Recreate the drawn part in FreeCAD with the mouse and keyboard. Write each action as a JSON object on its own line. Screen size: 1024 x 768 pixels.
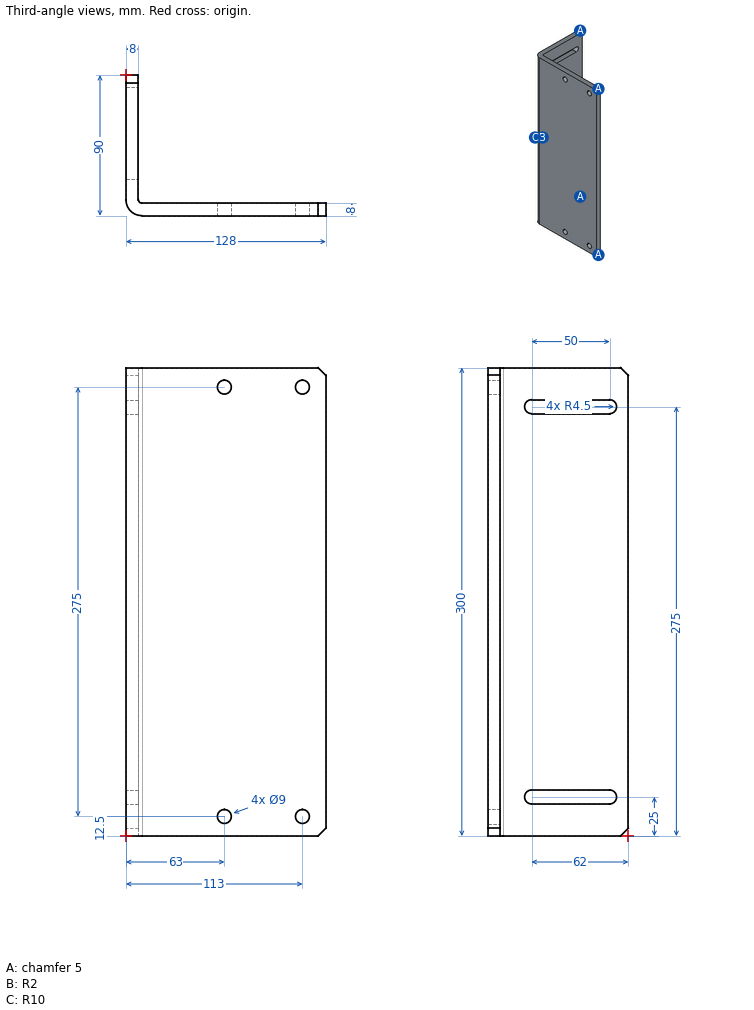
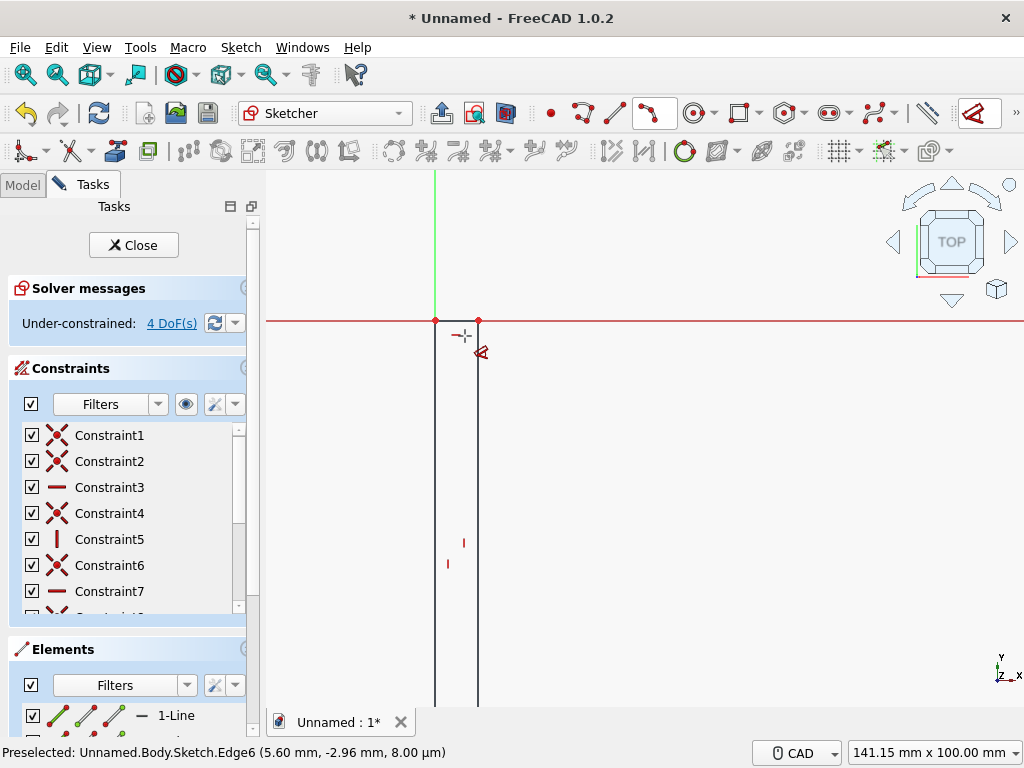
{"action": "scroll", "coordinate": [330, 288], "scroll_direction": "down", "scroll_amount": 3}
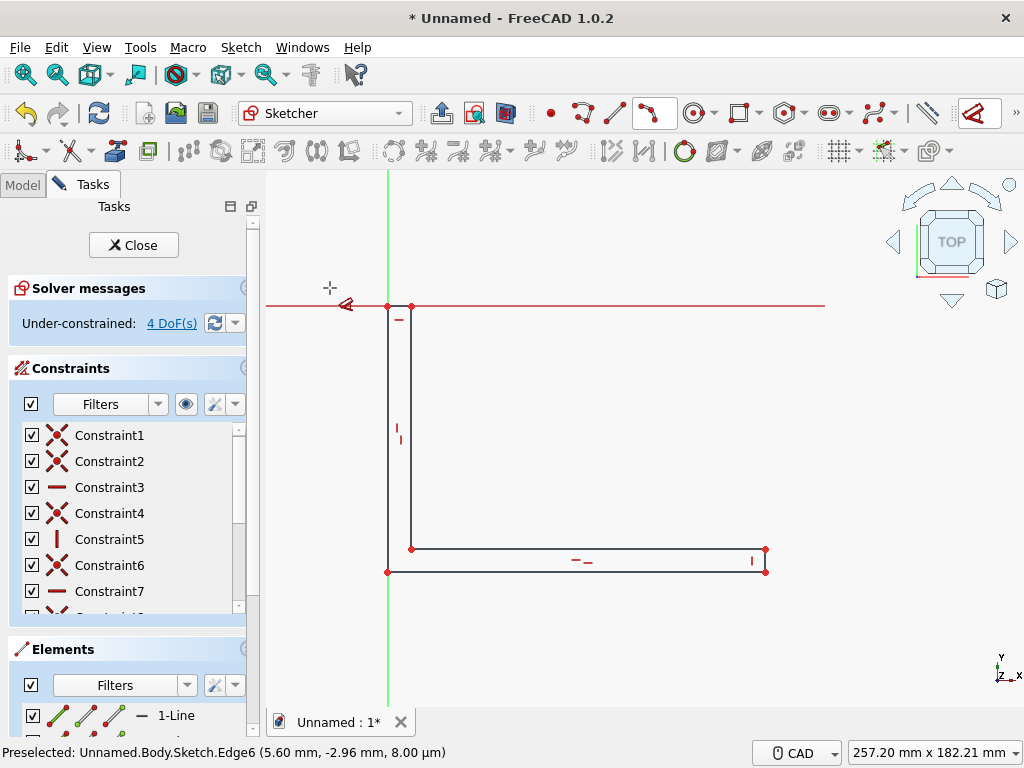
{"action": "scroll", "coordinate": [765, 566], "scroll_direction": "up", "scroll_amount": 4}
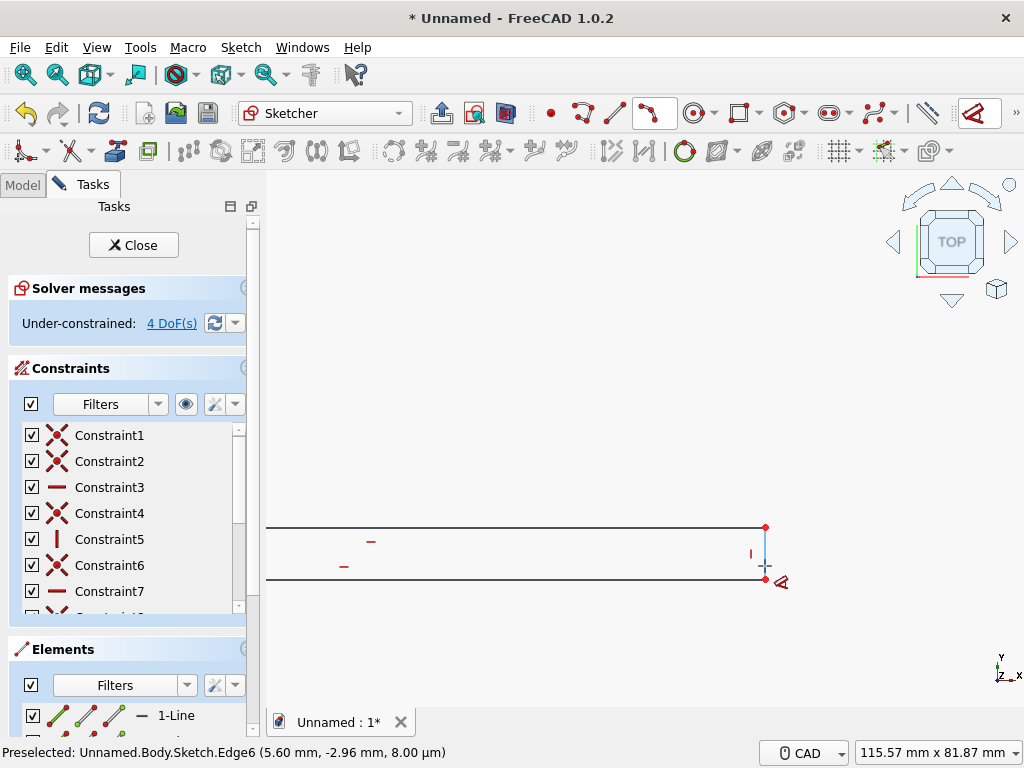
{"action": "left_click", "coordinate": [765, 564]}
{"action": "left_click", "coordinate": [799, 554]}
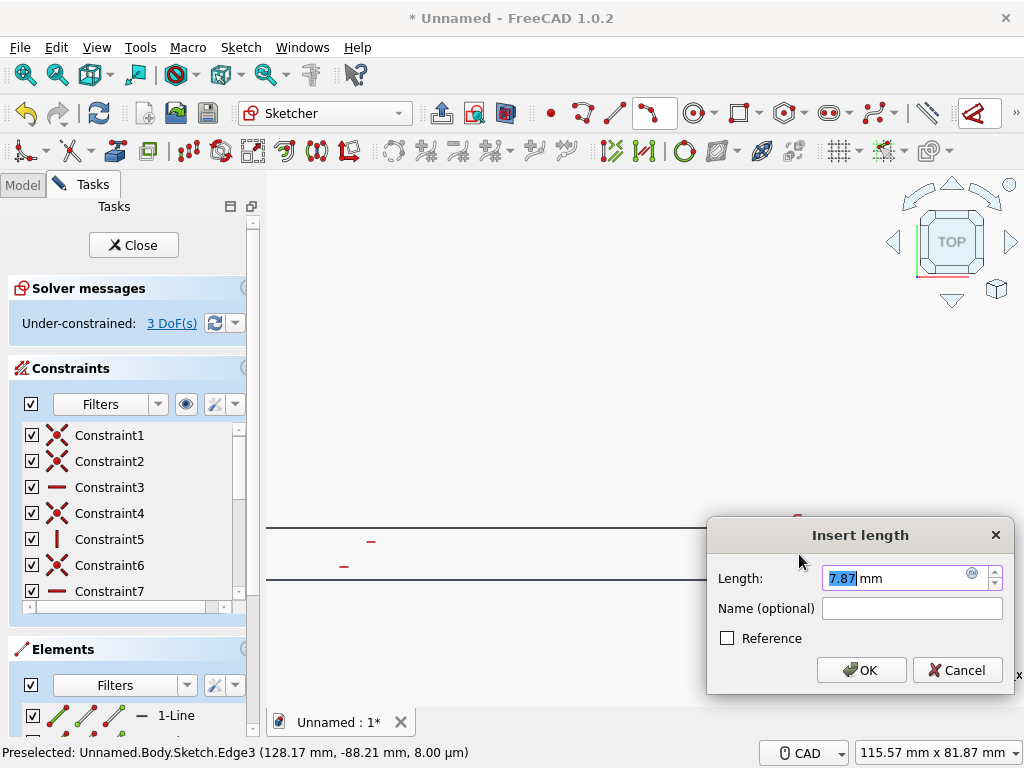
{"action": "type", "text": "8"}
{"action": "key", "text": "Return"}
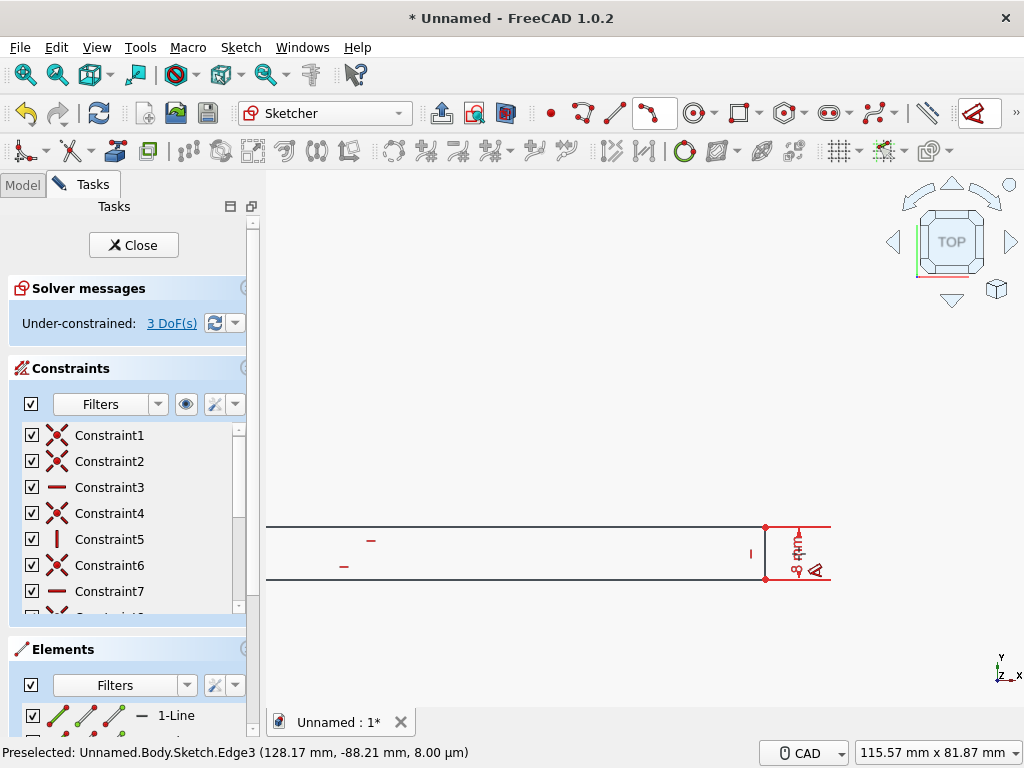
{"action": "scroll", "coordinate": [766, 567], "scroll_direction": "down", "scroll_amount": 4}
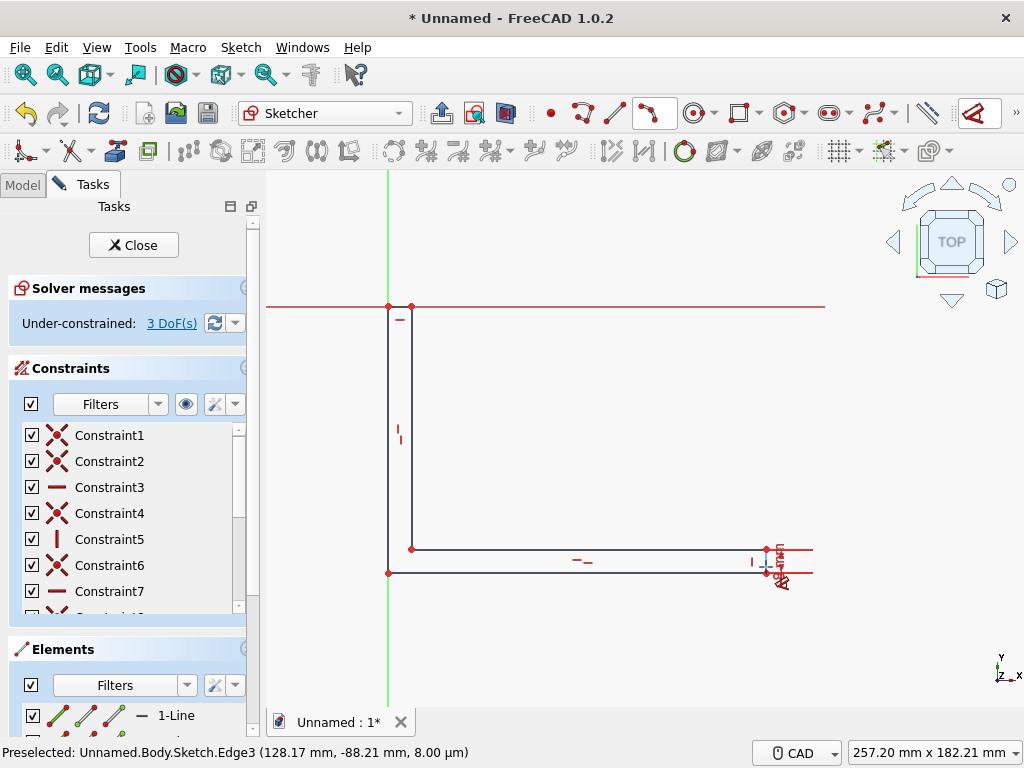
{"action": "scroll", "coordinate": [405, 307], "scroll_direction": "up", "scroll_amount": 4}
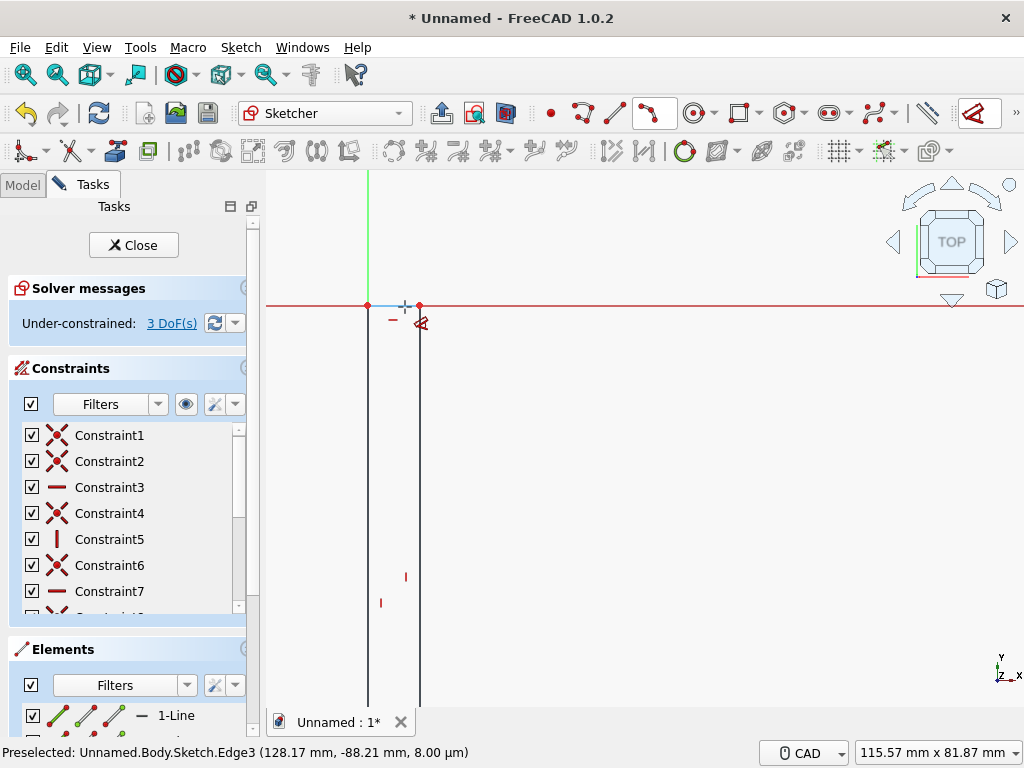
{"action": "left_click", "coordinate": [404, 306]}
{"action": "left_click", "coordinate": [394, 272]}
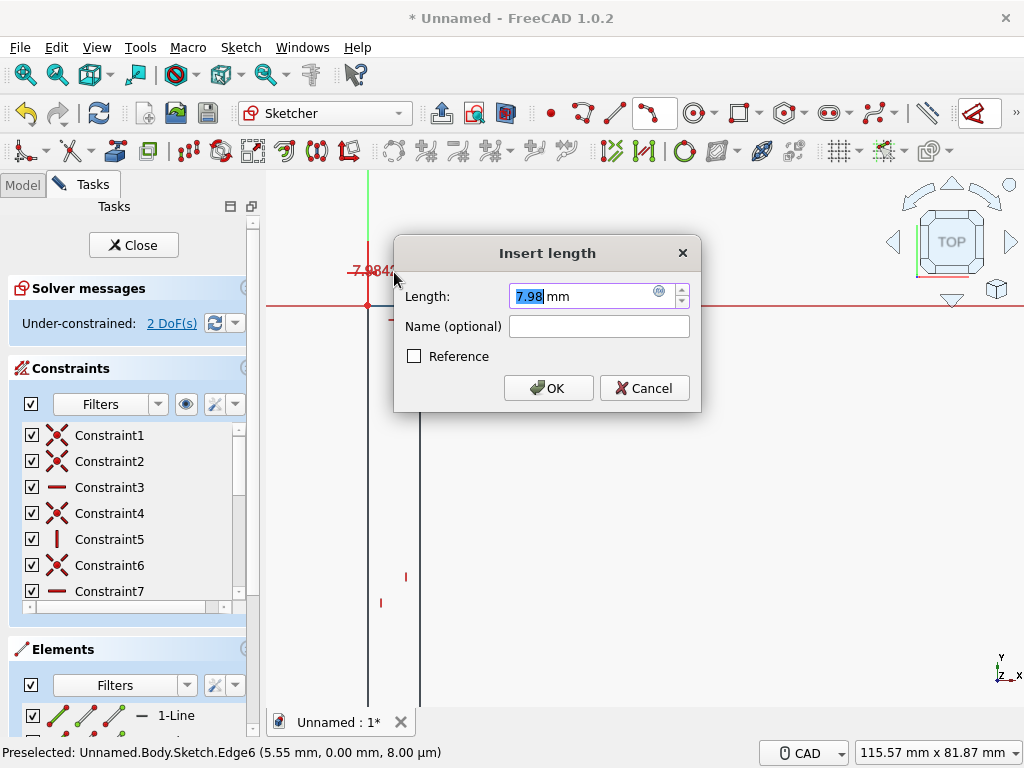
{"action": "type", "text": "8"}
{"action": "key", "text": "Return"}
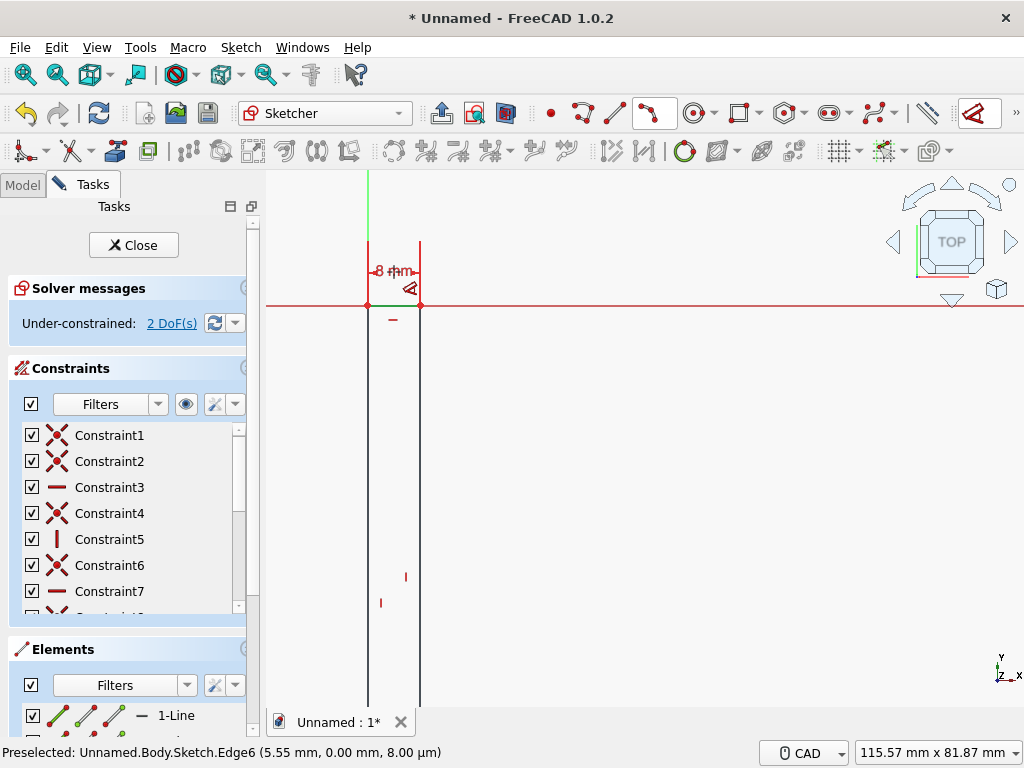
{"action": "left_click", "coordinate": [368, 484]}
{"action": "left_click", "coordinate": [334, 492]}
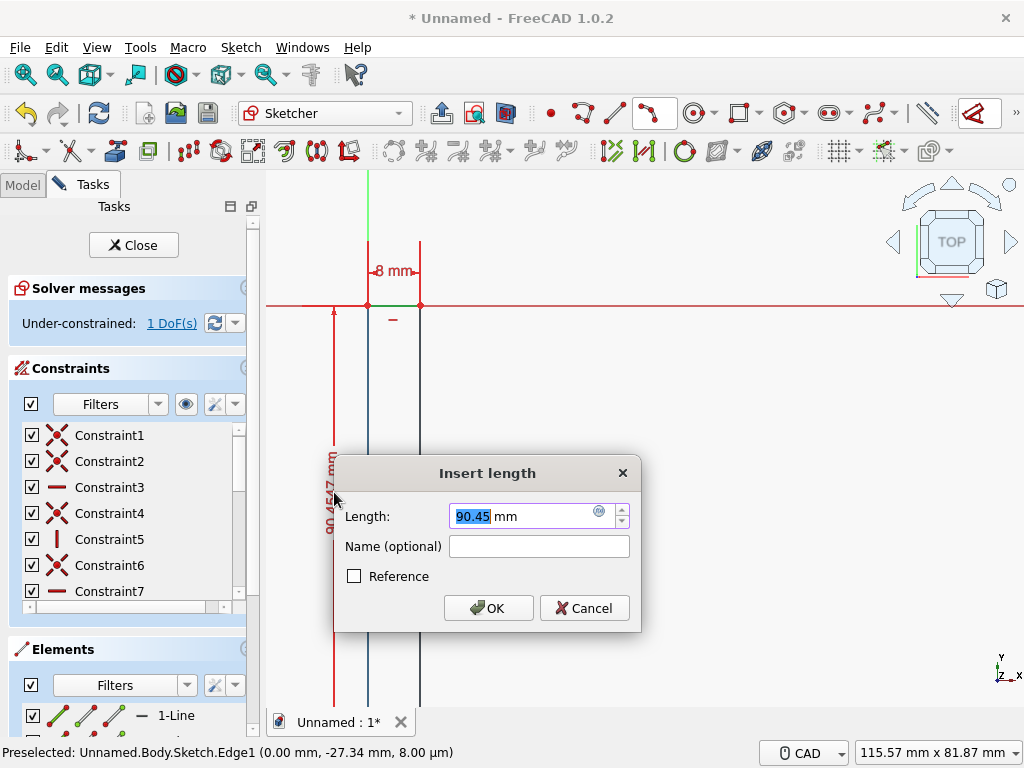
{"action": "type", "text": "90"}
{"action": "key", "text": "Return"}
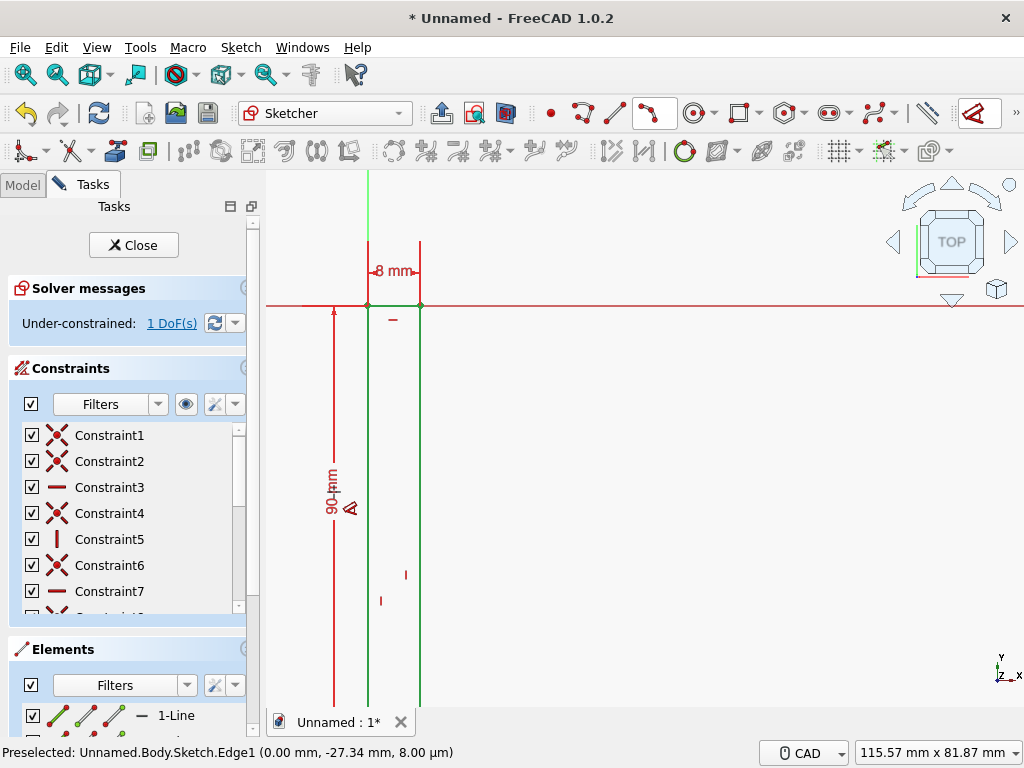
{"action": "scroll", "coordinate": [404, 306], "scroll_direction": "down", "scroll_amount": 4}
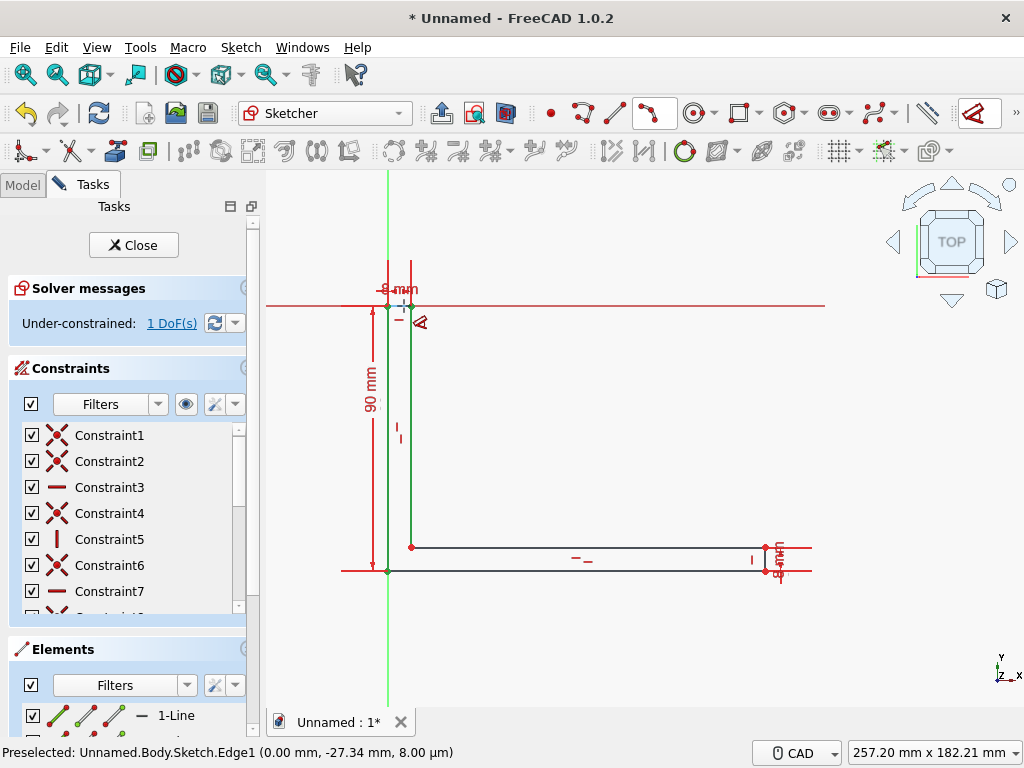
{"action": "left_click", "coordinate": [501, 571]}
{"action": "left_click", "coordinate": [577, 605]}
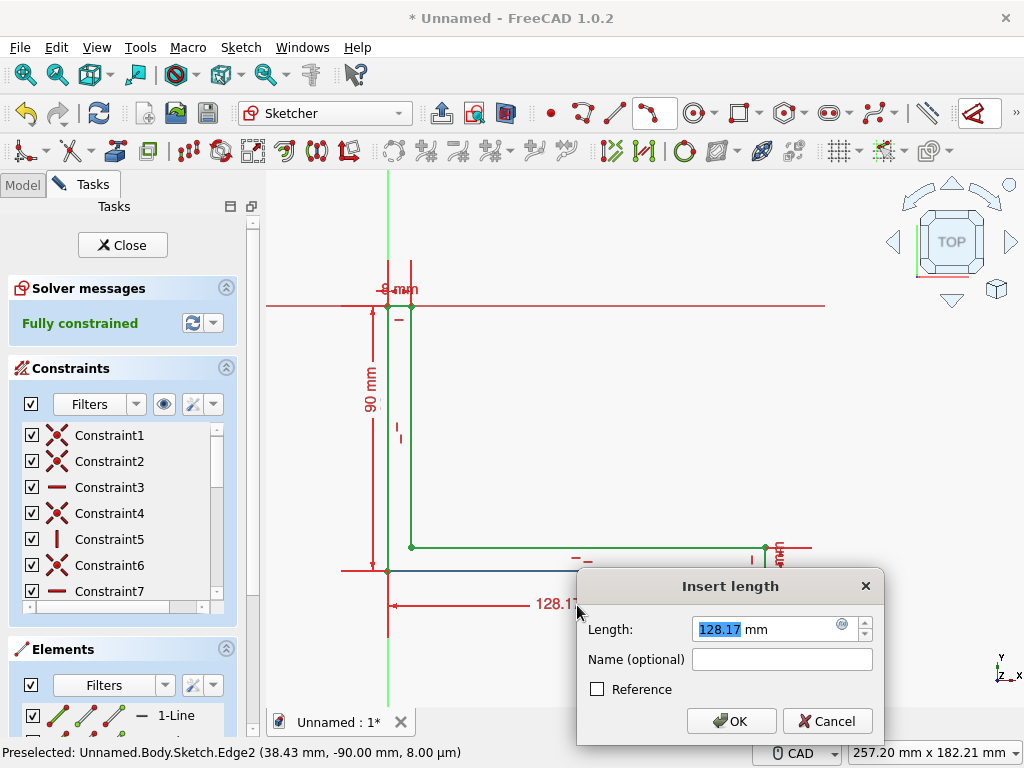
{"action": "type", "text": "128"}
{"action": "key", "text": "Return"}
{"action": "key", "text": "Escape"}